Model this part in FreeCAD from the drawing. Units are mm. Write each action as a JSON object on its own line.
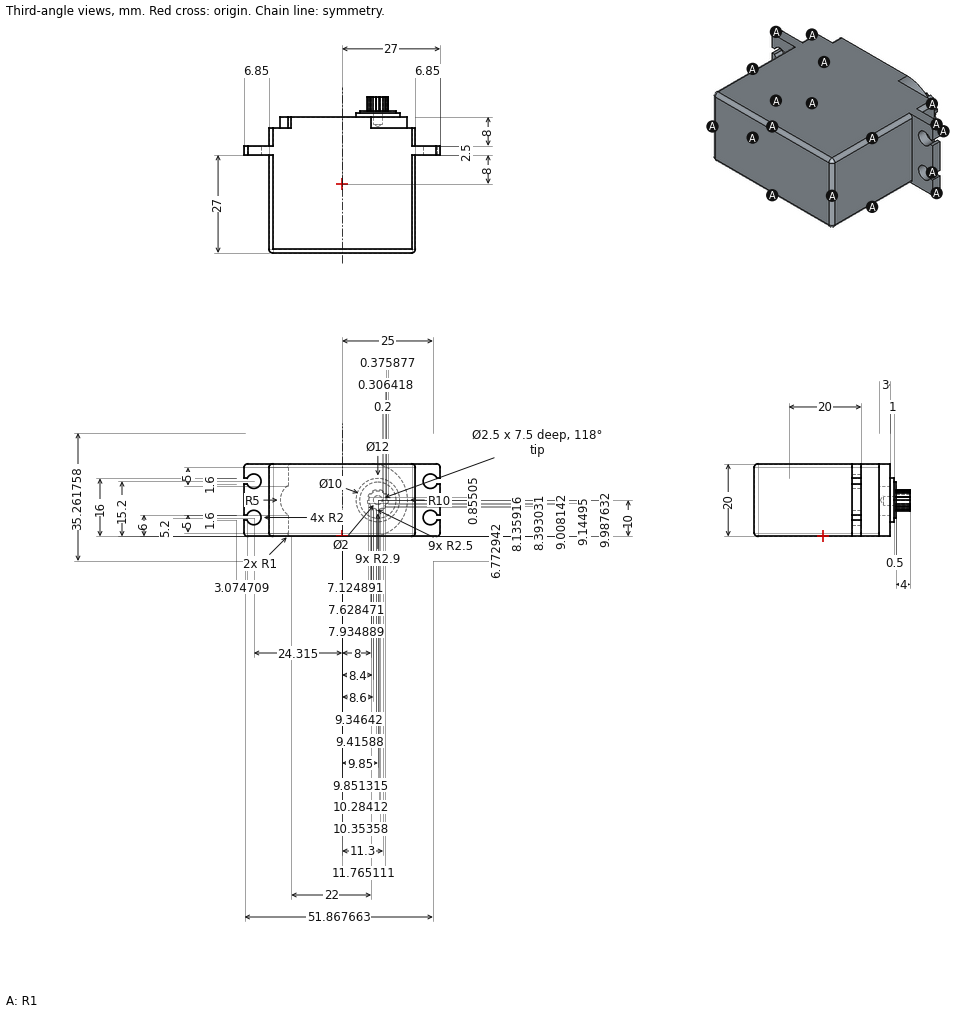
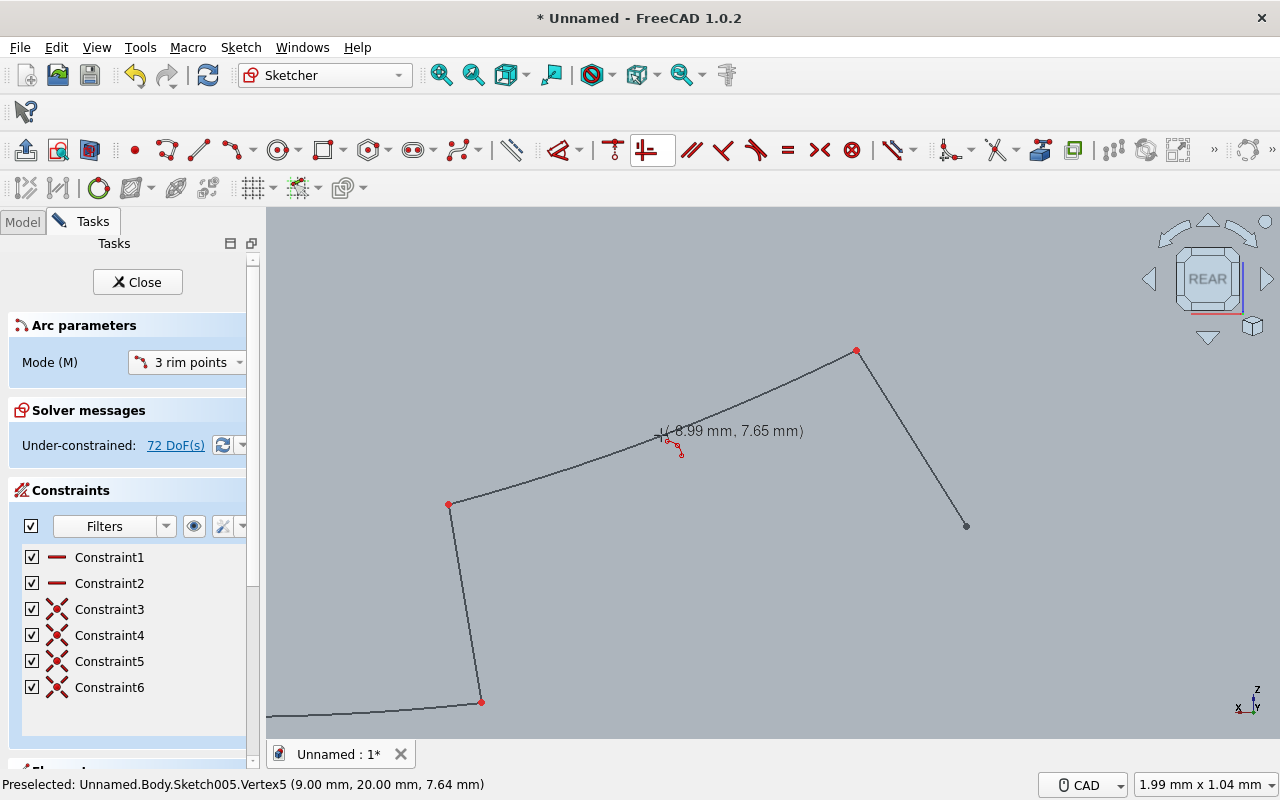
{"action": "scroll", "coordinate": [637, 442], "scroll_direction": "down", "scroll_amount": 15}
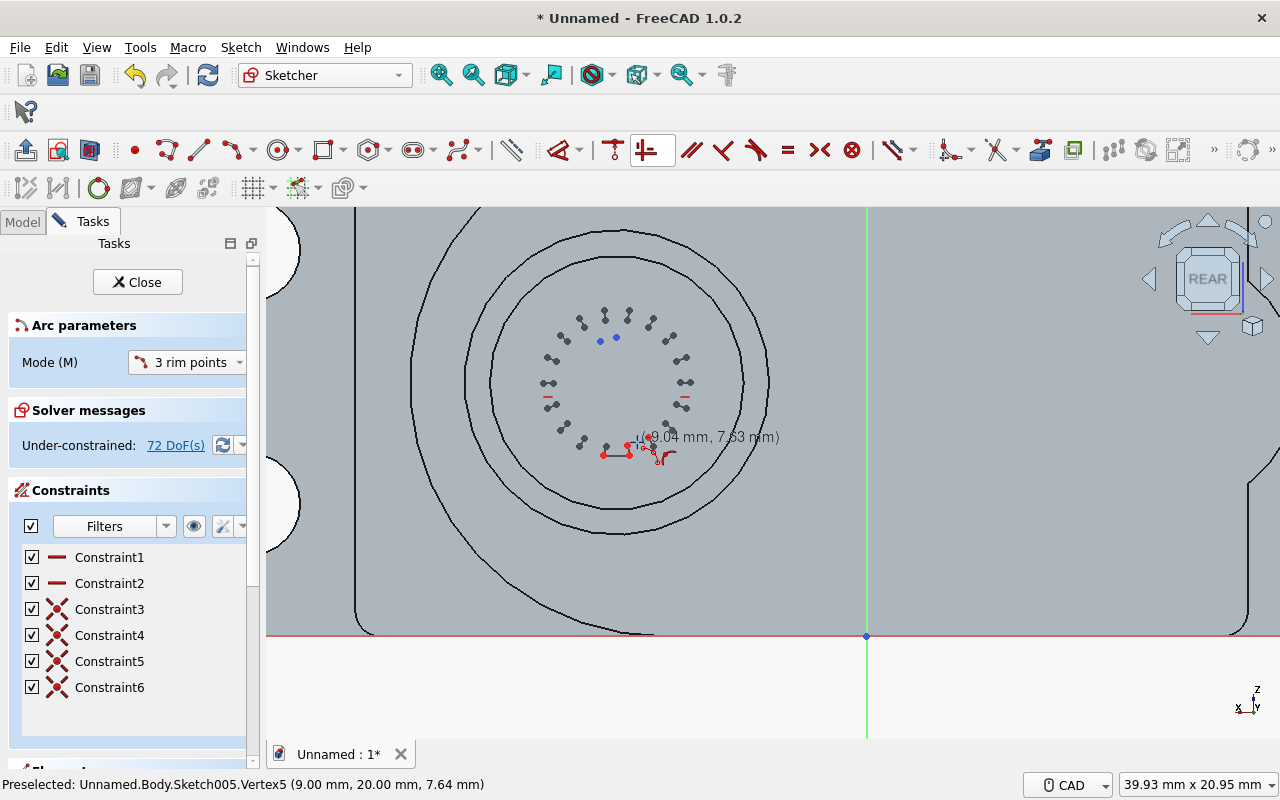
{"action": "scroll", "coordinate": [654, 446], "scroll_direction": "up", "scroll_amount": 6}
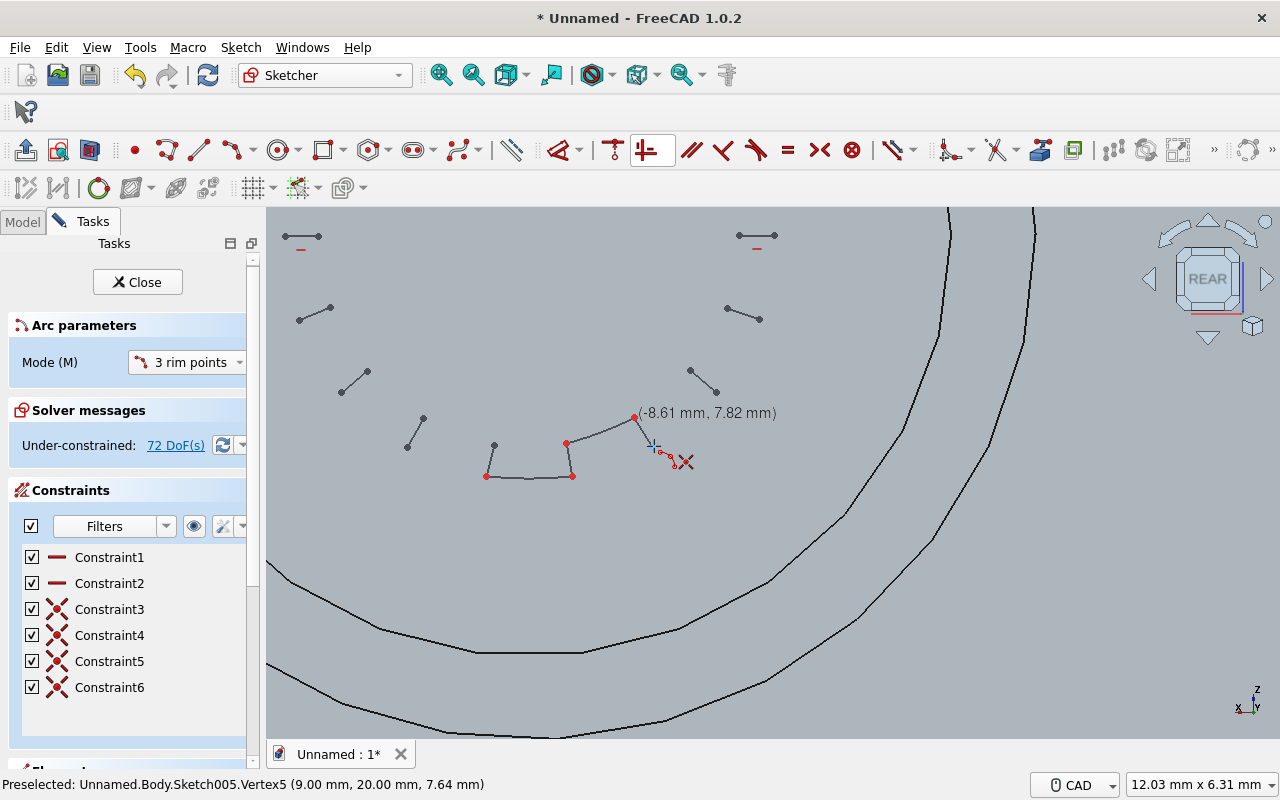
{"action": "left_click", "coordinate": [652, 447]}
{"action": "left_click", "coordinate": [716, 392]}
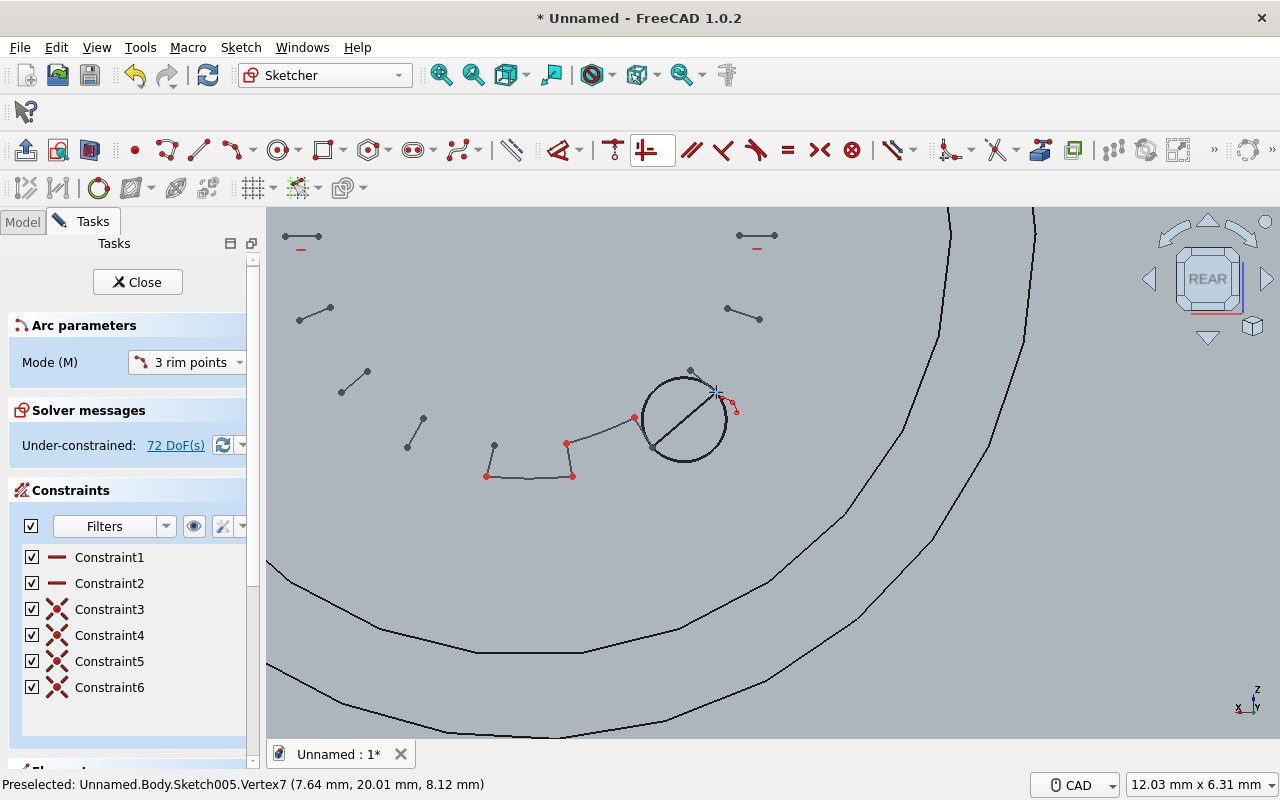
{"action": "scroll", "coordinate": [687, 421], "scroll_direction": "up", "scroll_amount": 8}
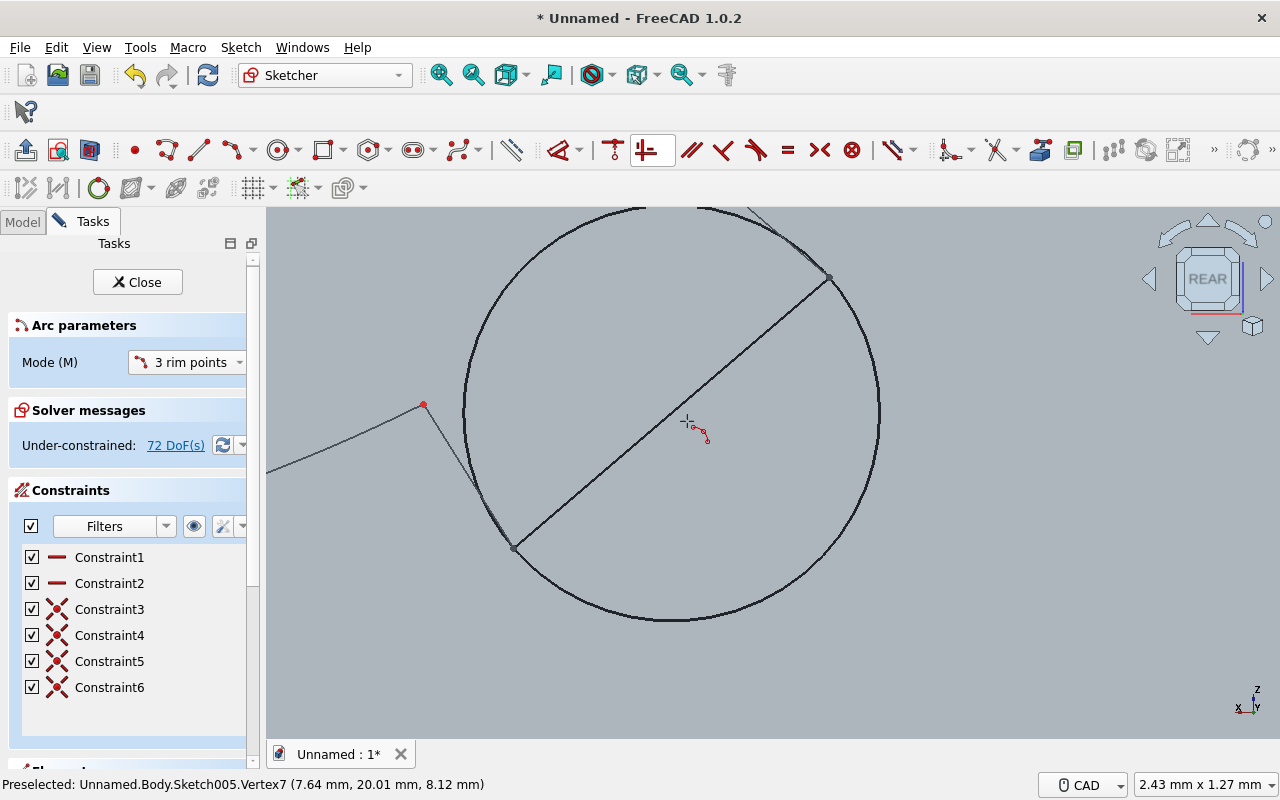
{"action": "left_click", "coordinate": [684, 420]}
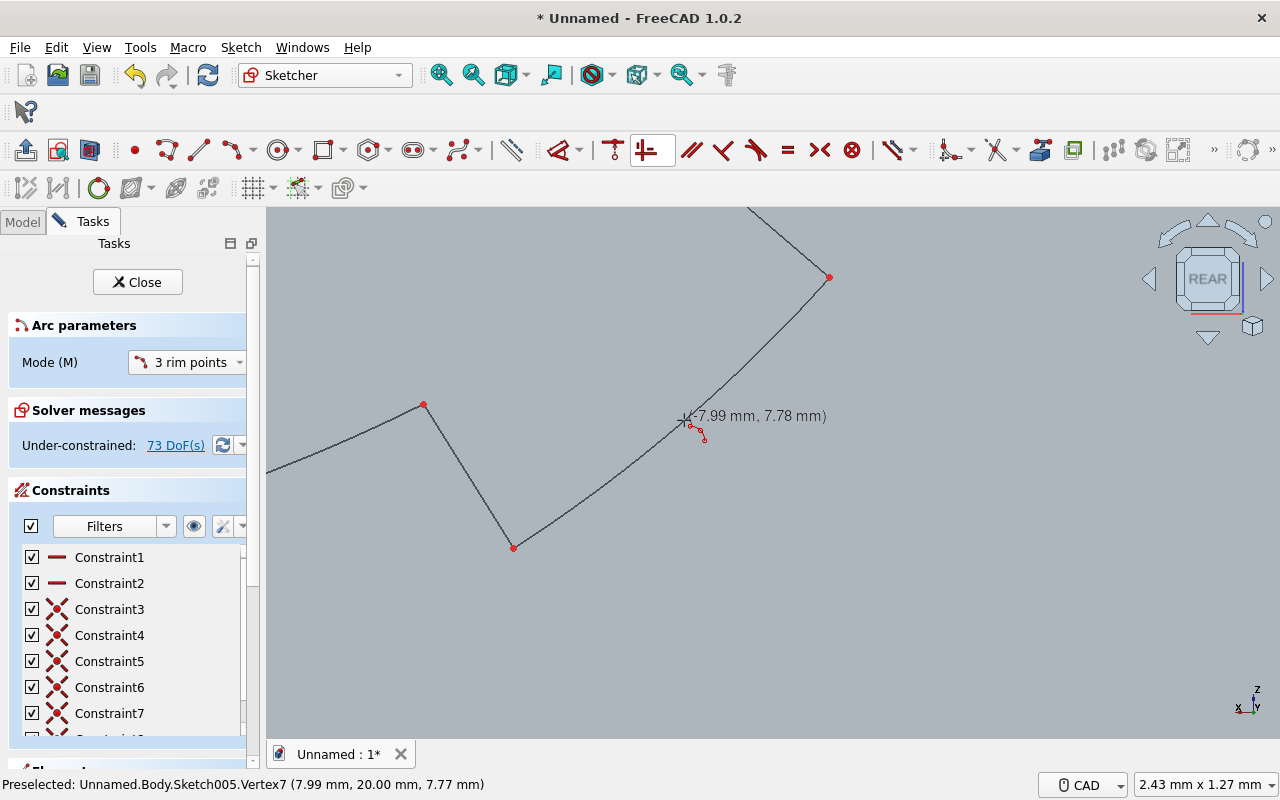
{"action": "scroll", "coordinate": [662, 440], "scroll_direction": "down", "scroll_amount": 14}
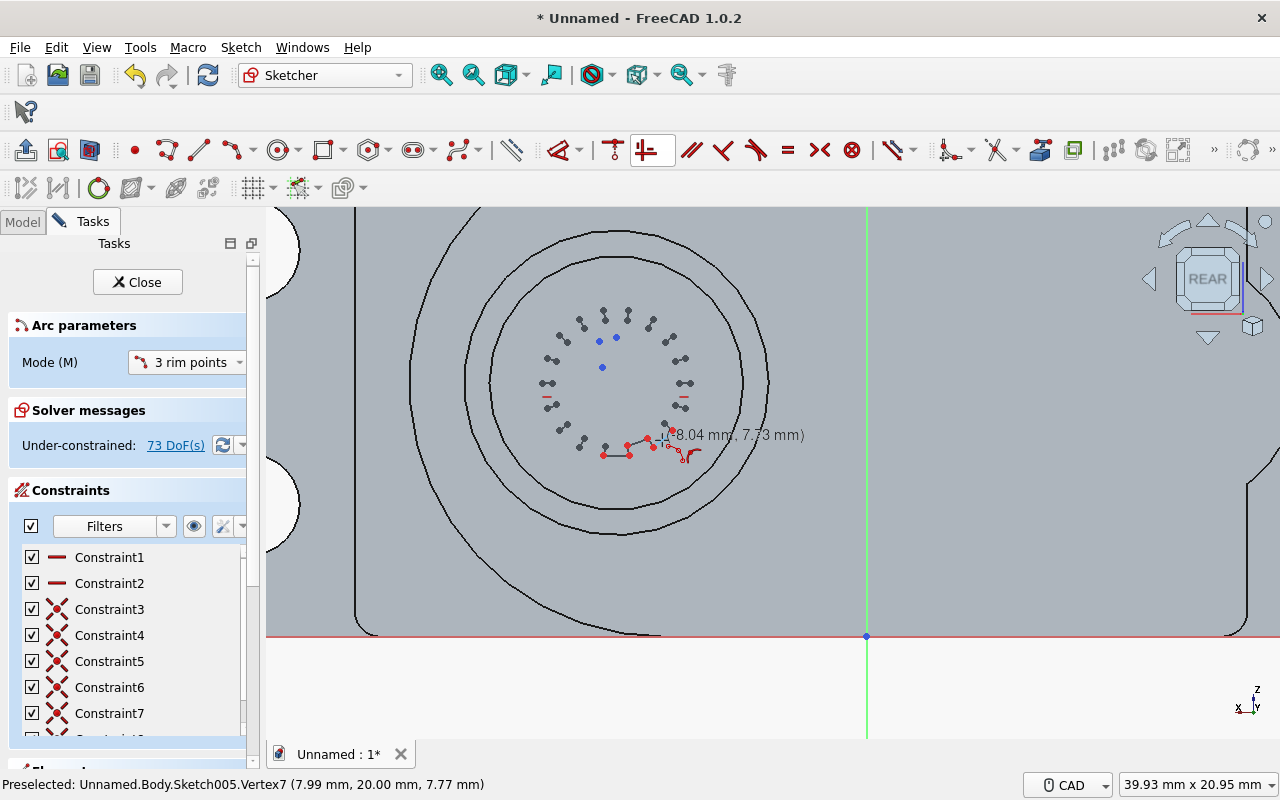
{"action": "scroll", "coordinate": [665, 424], "scroll_direction": "up", "scroll_amount": 6}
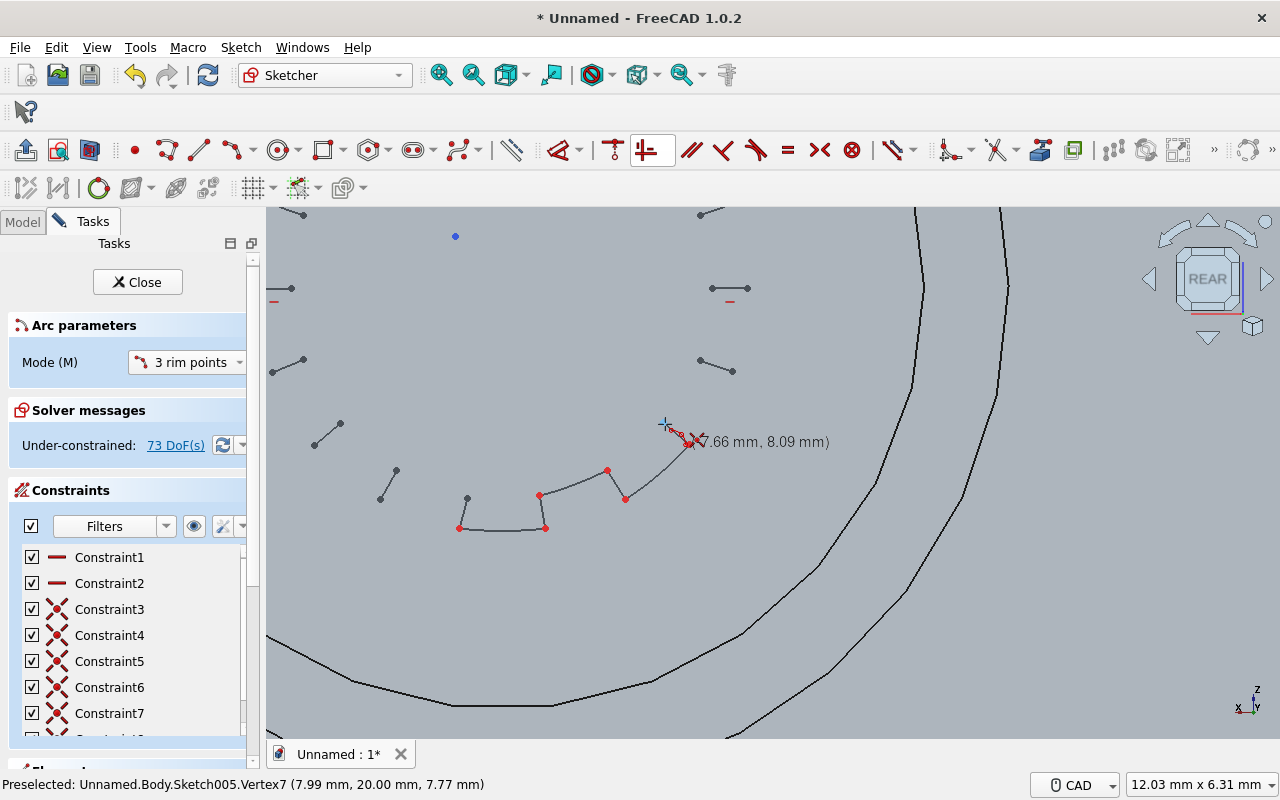
{"action": "left_click", "coordinate": [664, 423]}
{"action": "left_click", "coordinate": [700, 361]}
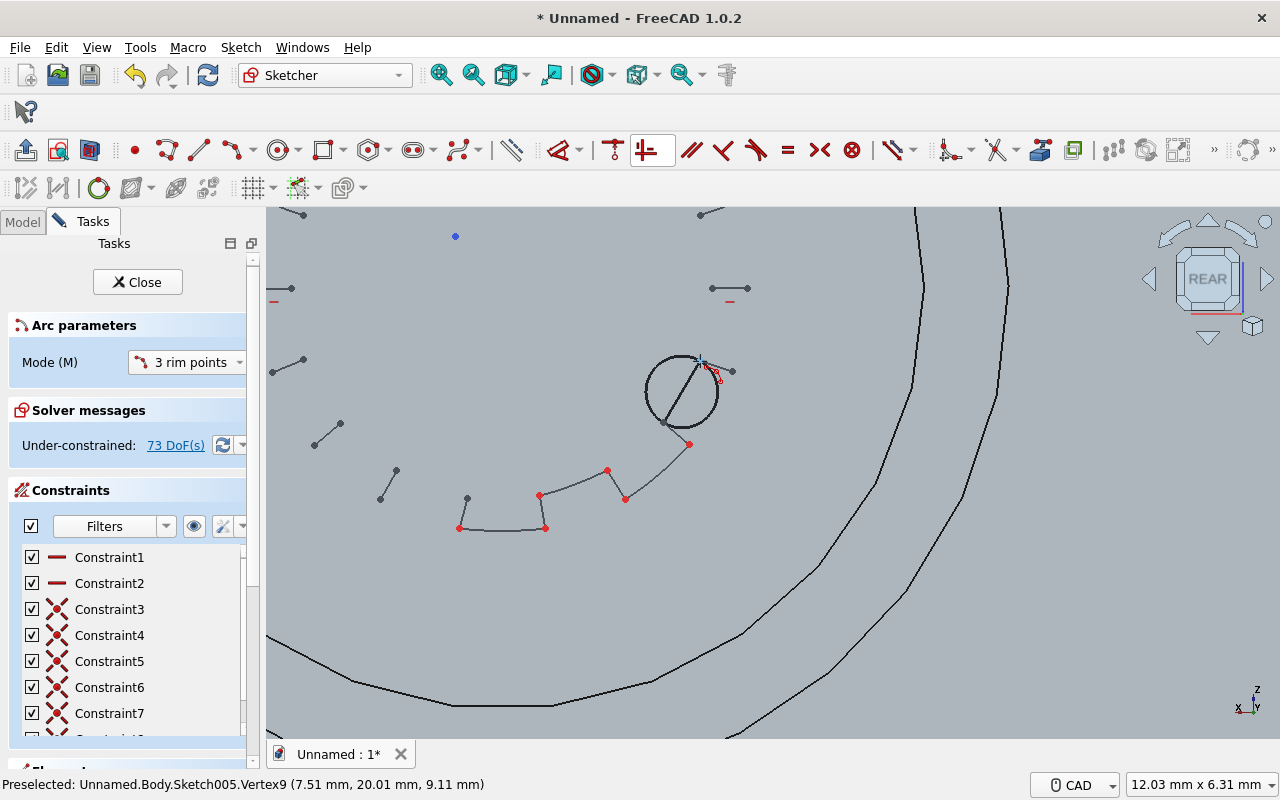
{"action": "scroll", "coordinate": [685, 392], "scroll_direction": "up", "scroll_amount": 9}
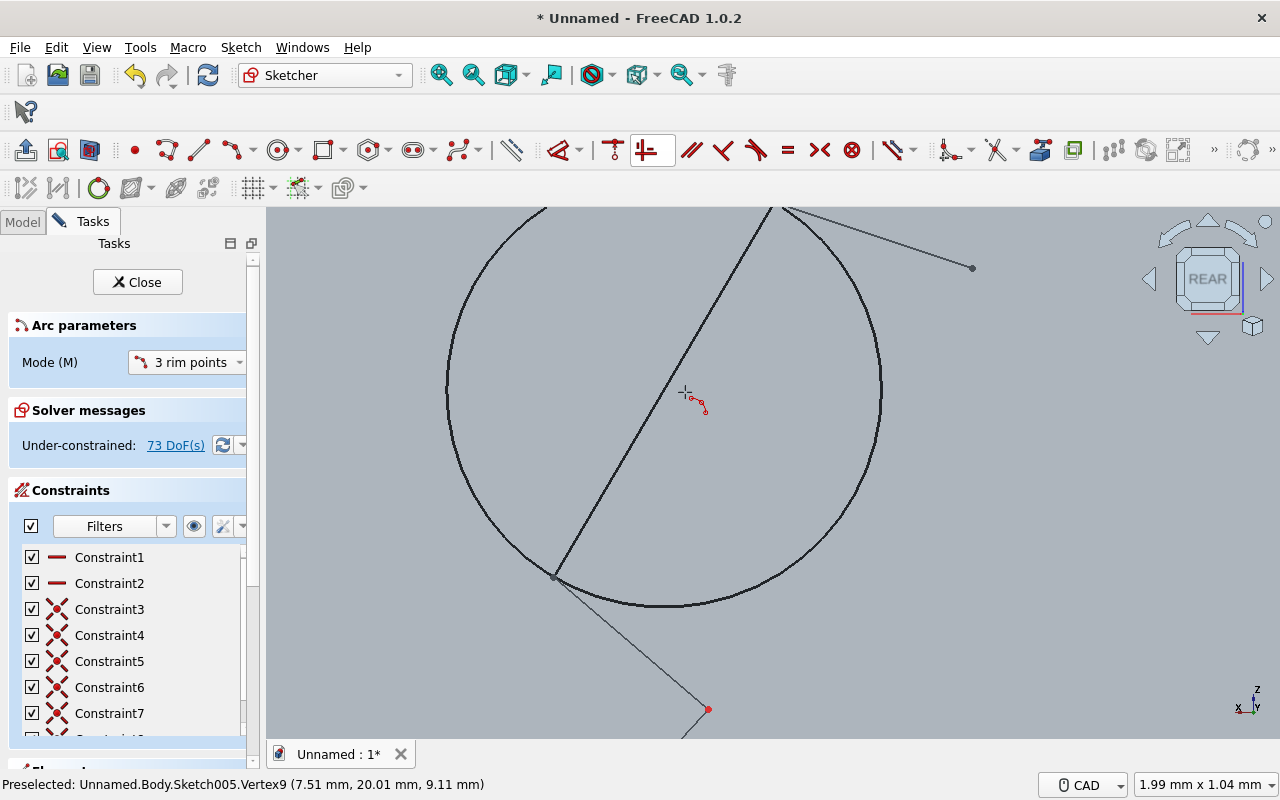
{"action": "left_click", "coordinate": [684, 387]}